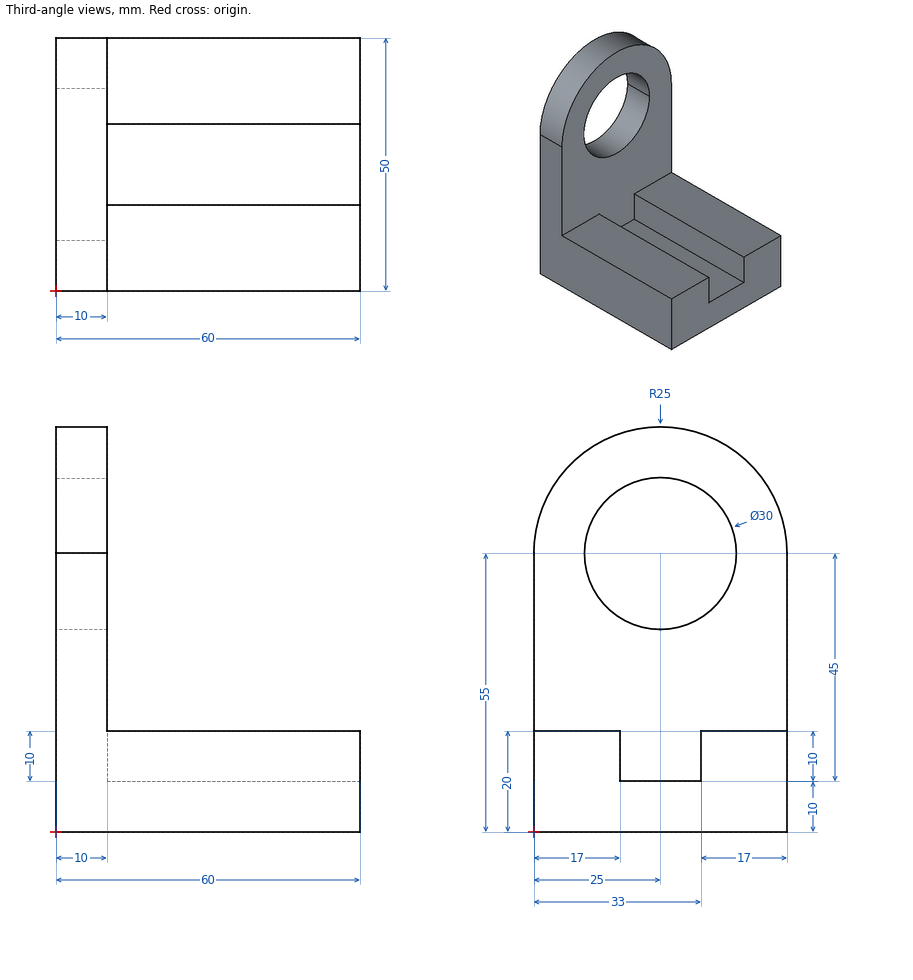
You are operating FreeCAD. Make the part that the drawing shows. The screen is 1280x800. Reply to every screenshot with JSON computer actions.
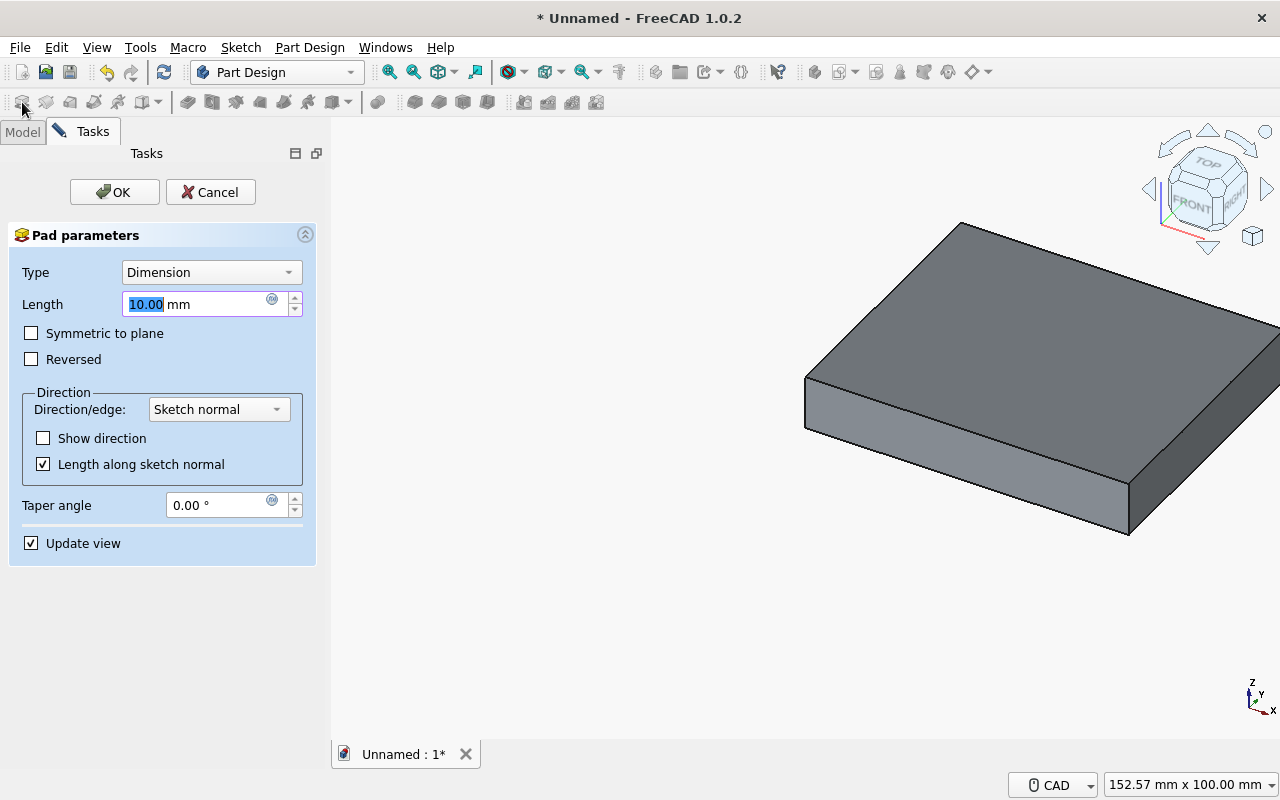
{"action": "type", "text": "60"}
{"action": "key", "text": "Tab"}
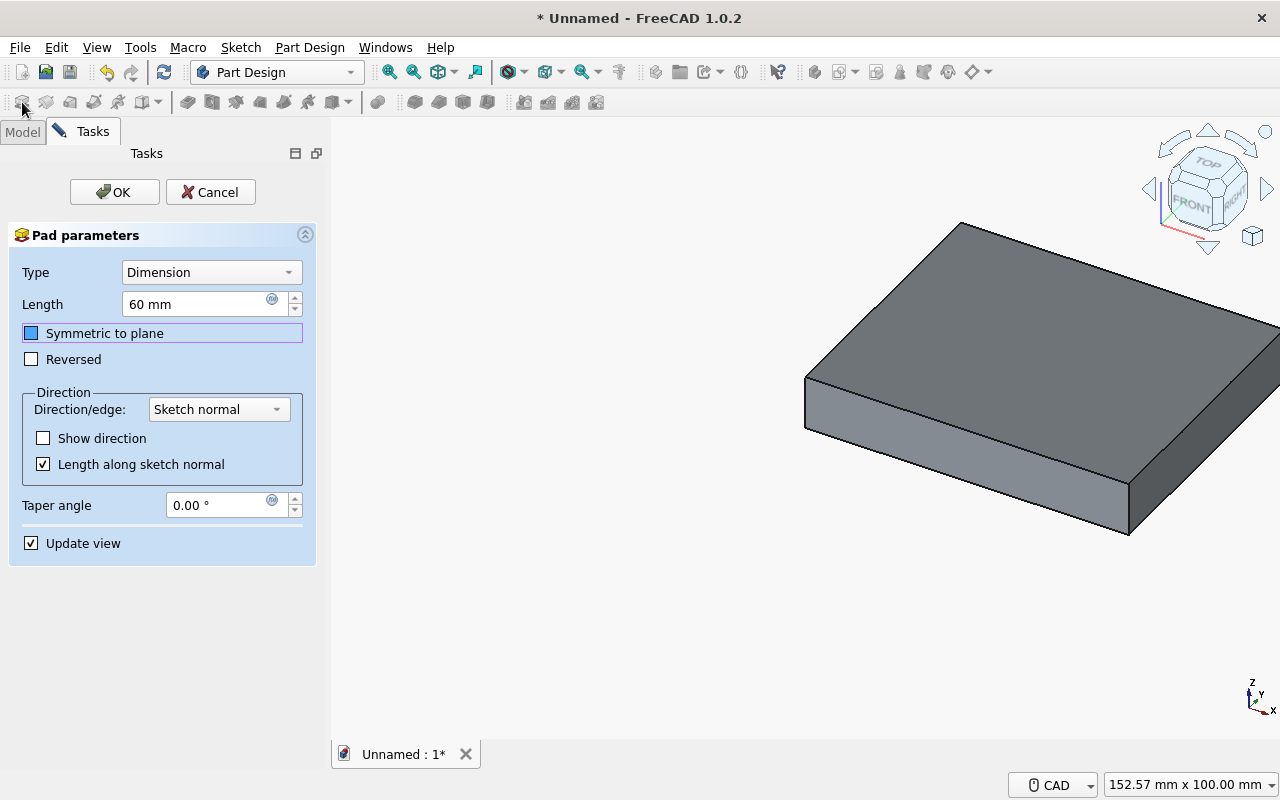
{"action": "left_click", "coordinate": [30, 359]}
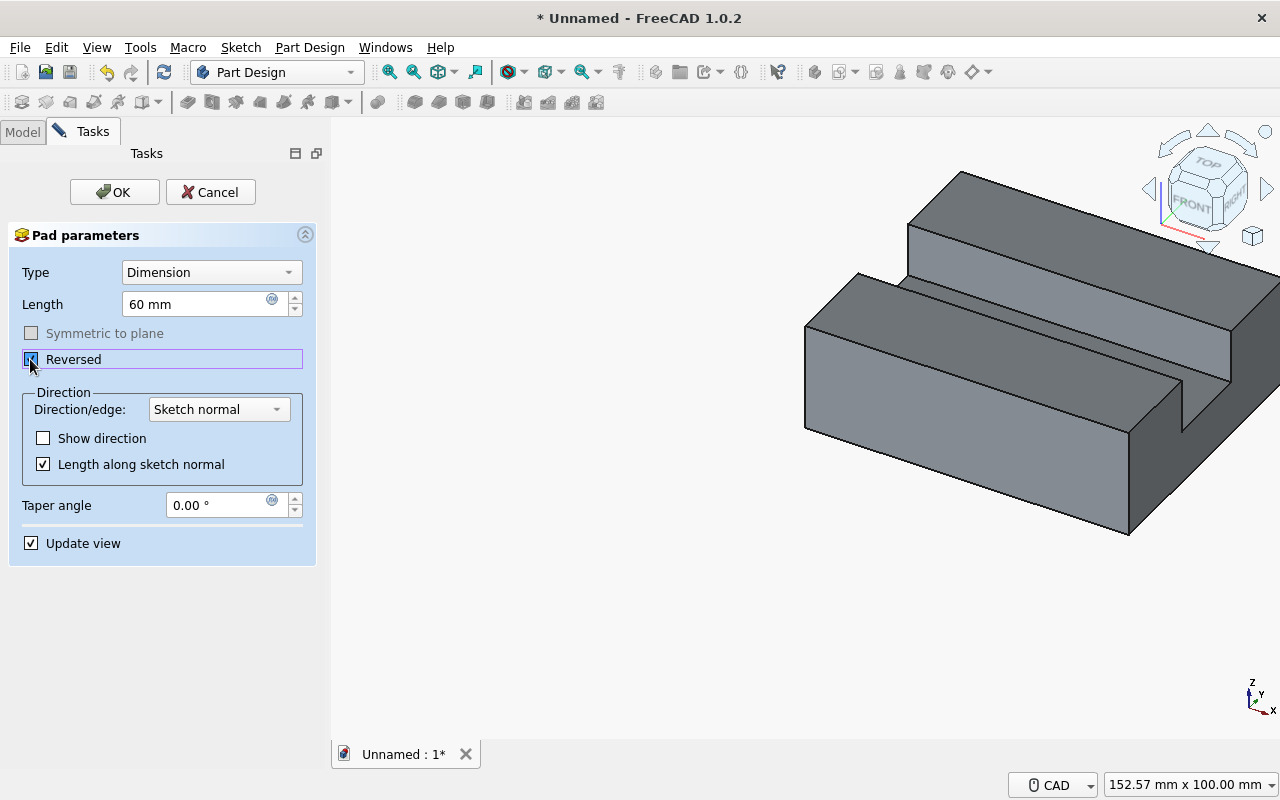
{"action": "left_click", "coordinate": [115, 192]}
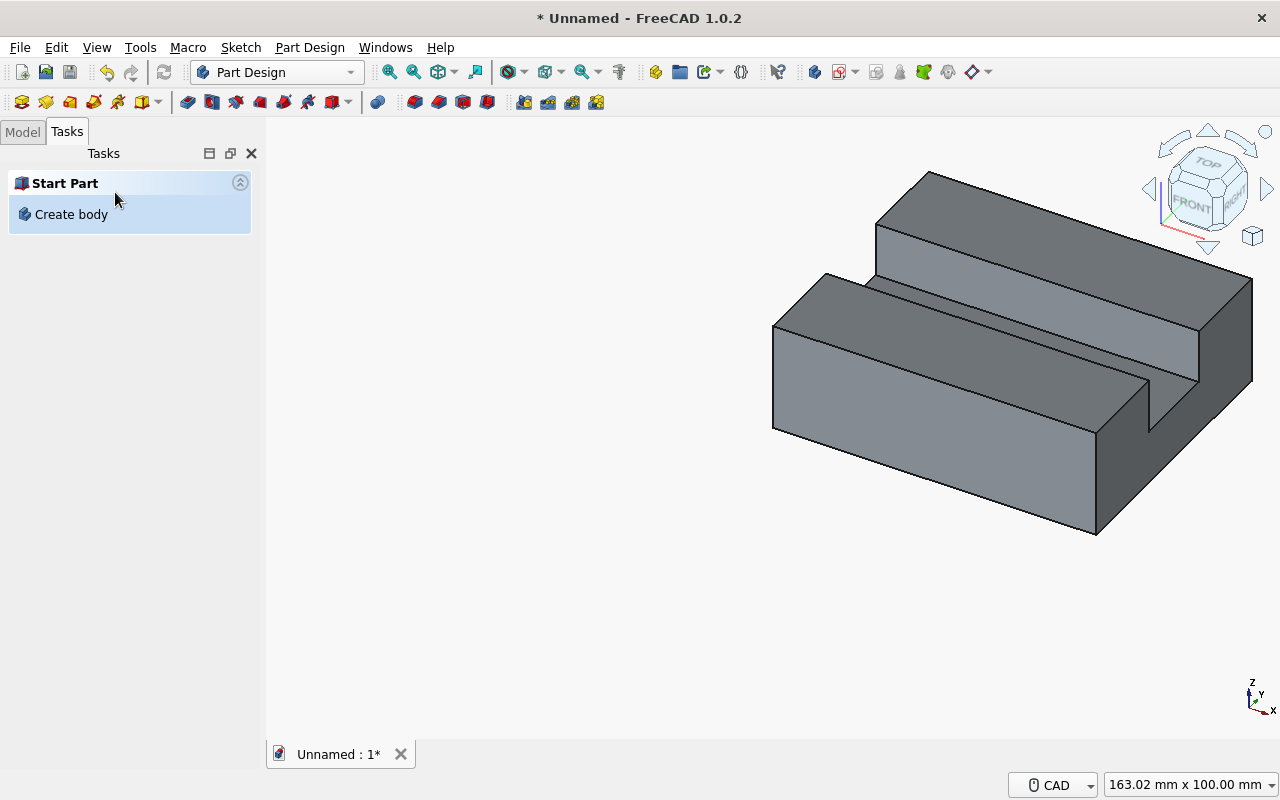
{"action": "left_click", "coordinate": [1053, 383]}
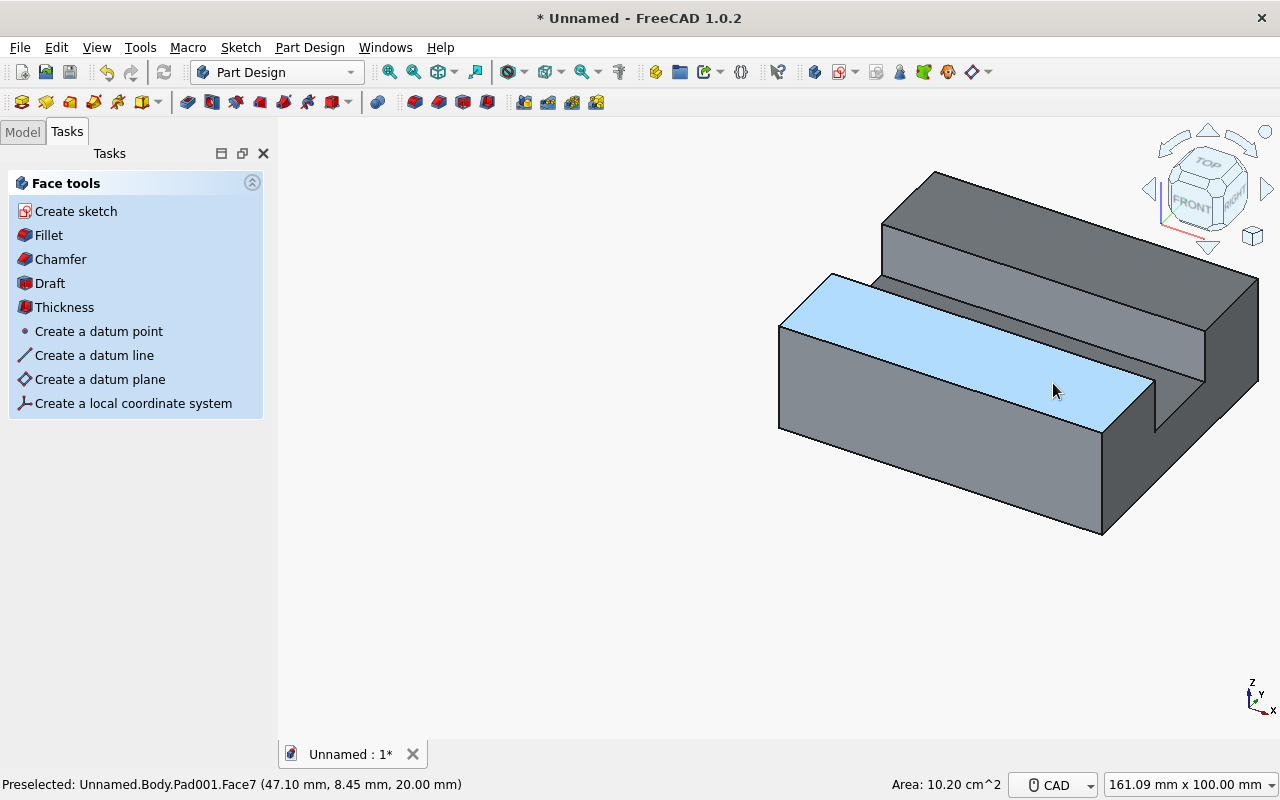
{"action": "left_click", "coordinate": [840, 72]}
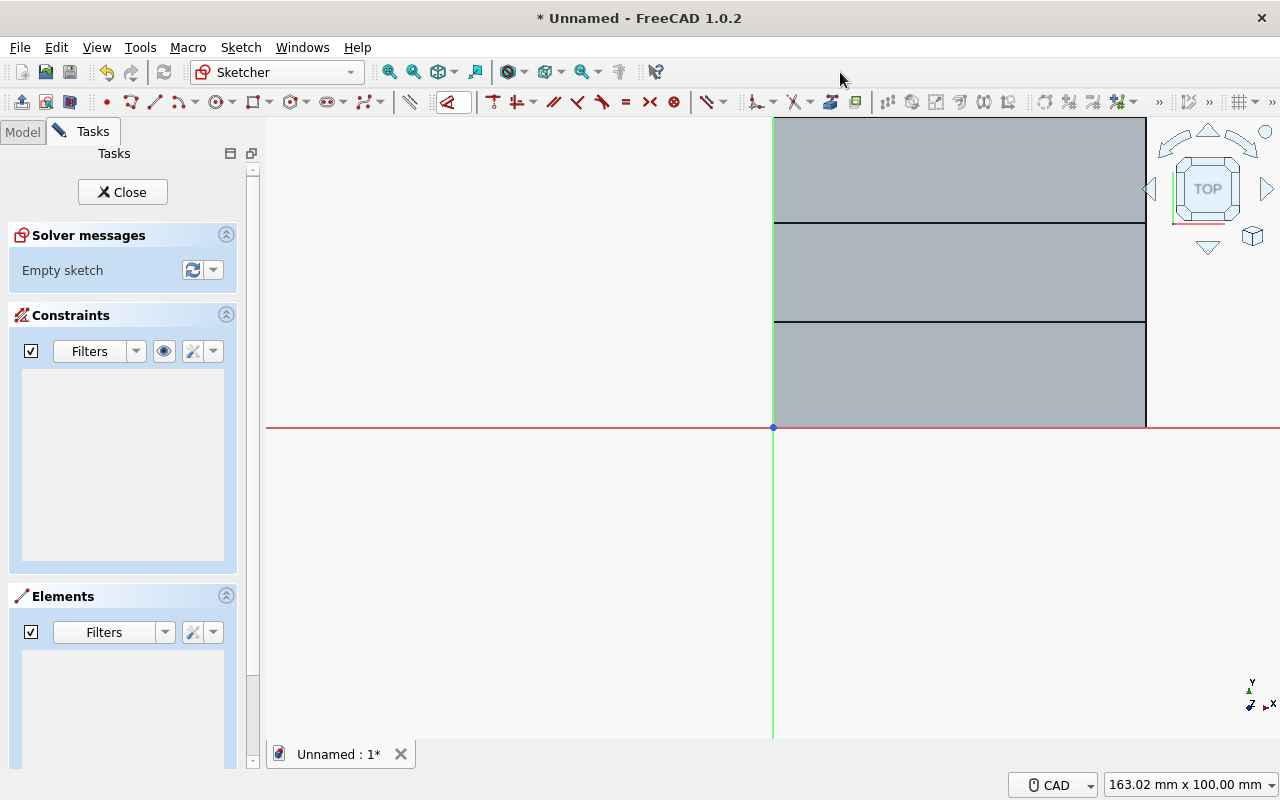
{"action": "scroll", "coordinate": [294, 711], "scroll_direction": "down", "scroll_amount": 1}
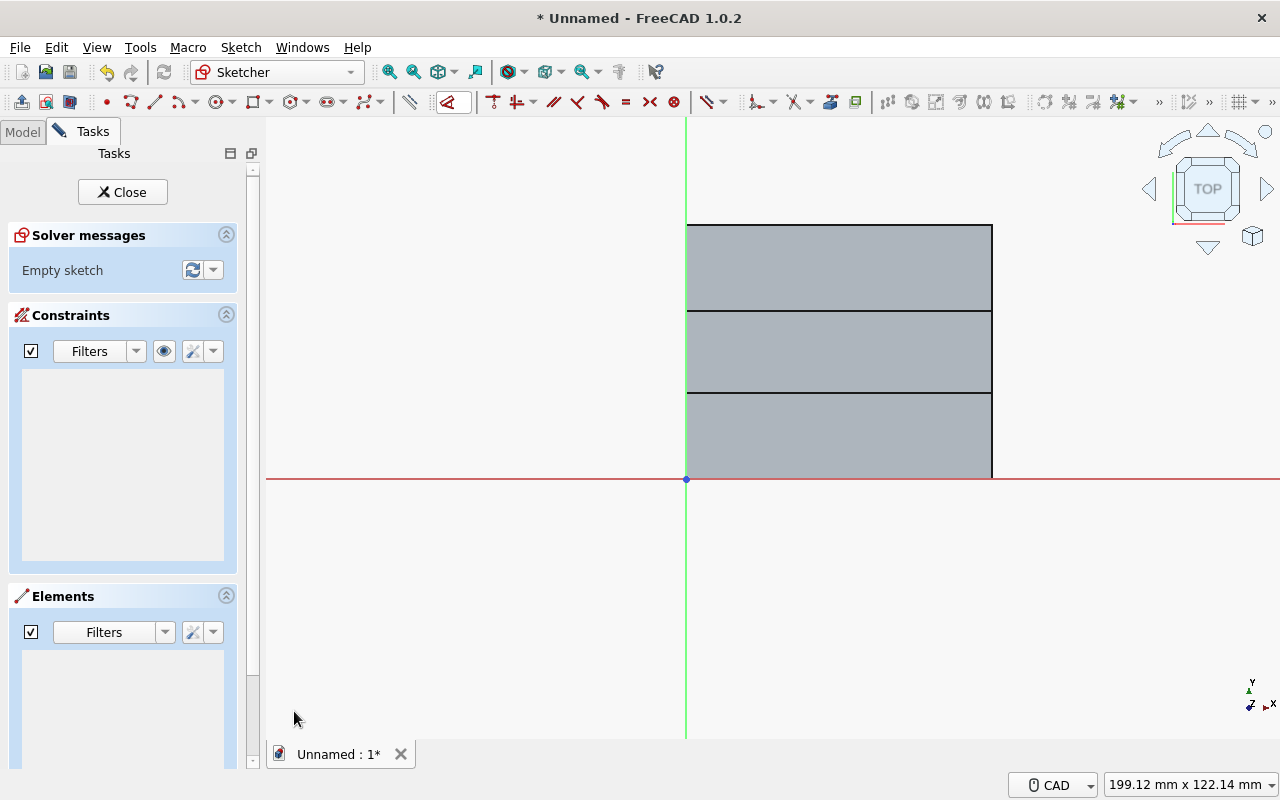
{"action": "scroll", "coordinate": [726, 198], "scroll_direction": "up", "scroll_amount": 2}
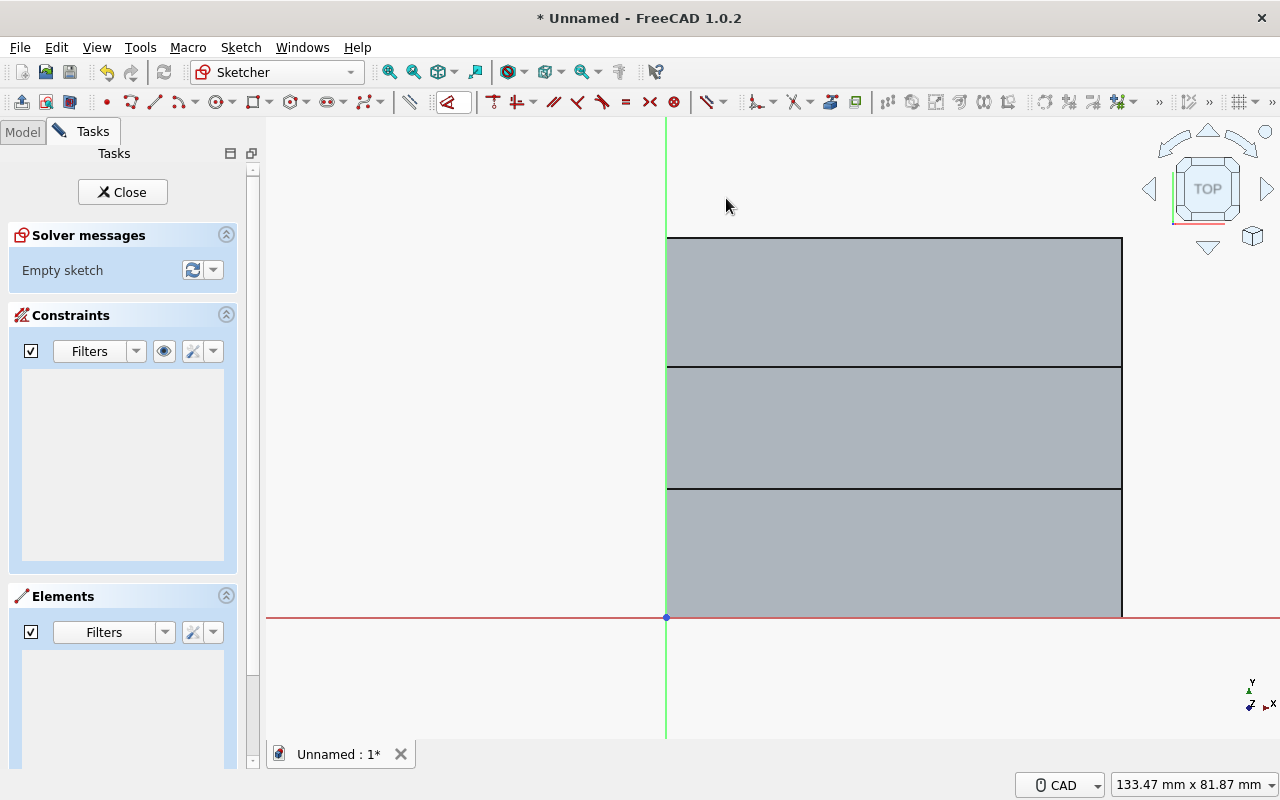
{"action": "left_click", "coordinate": [254, 102]}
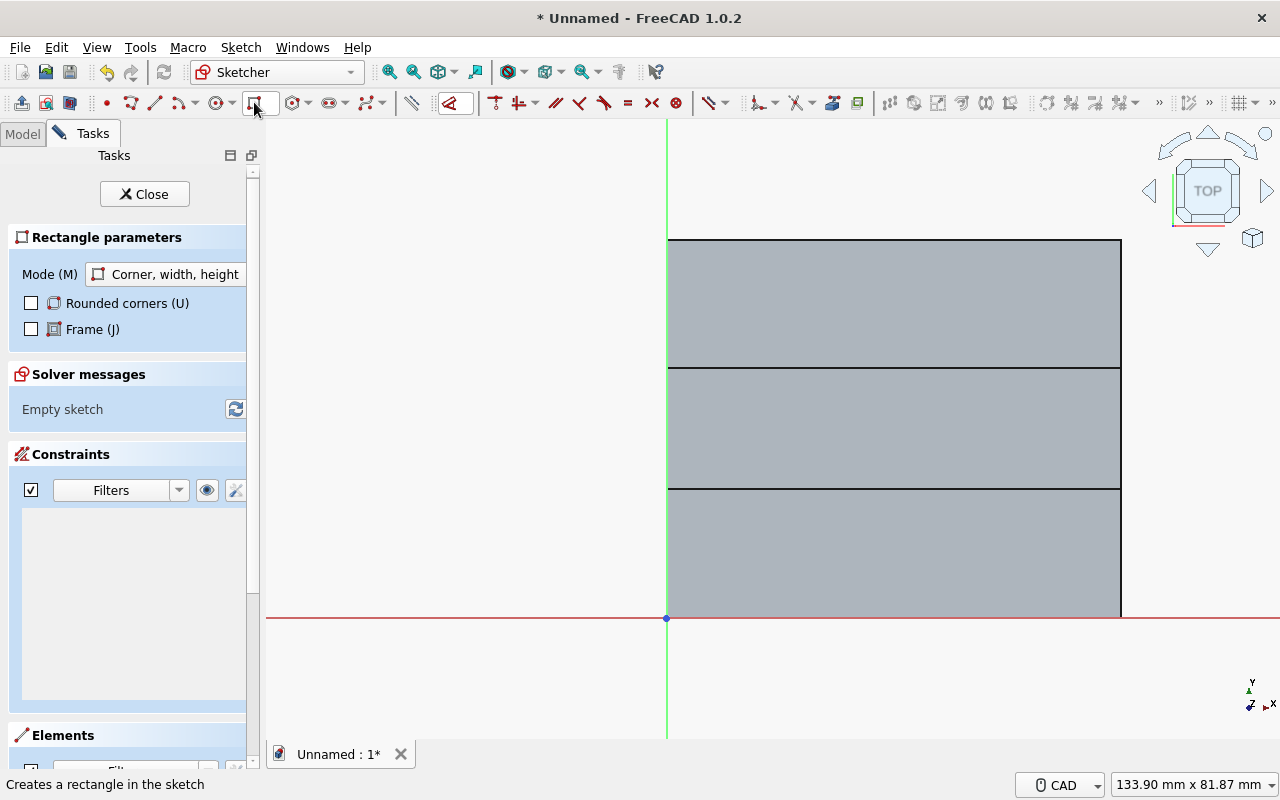
{"action": "left_click", "coordinate": [667, 618]}
{"action": "left_click", "coordinate": [742, 240]}
{"action": "key", "text": "Escape"}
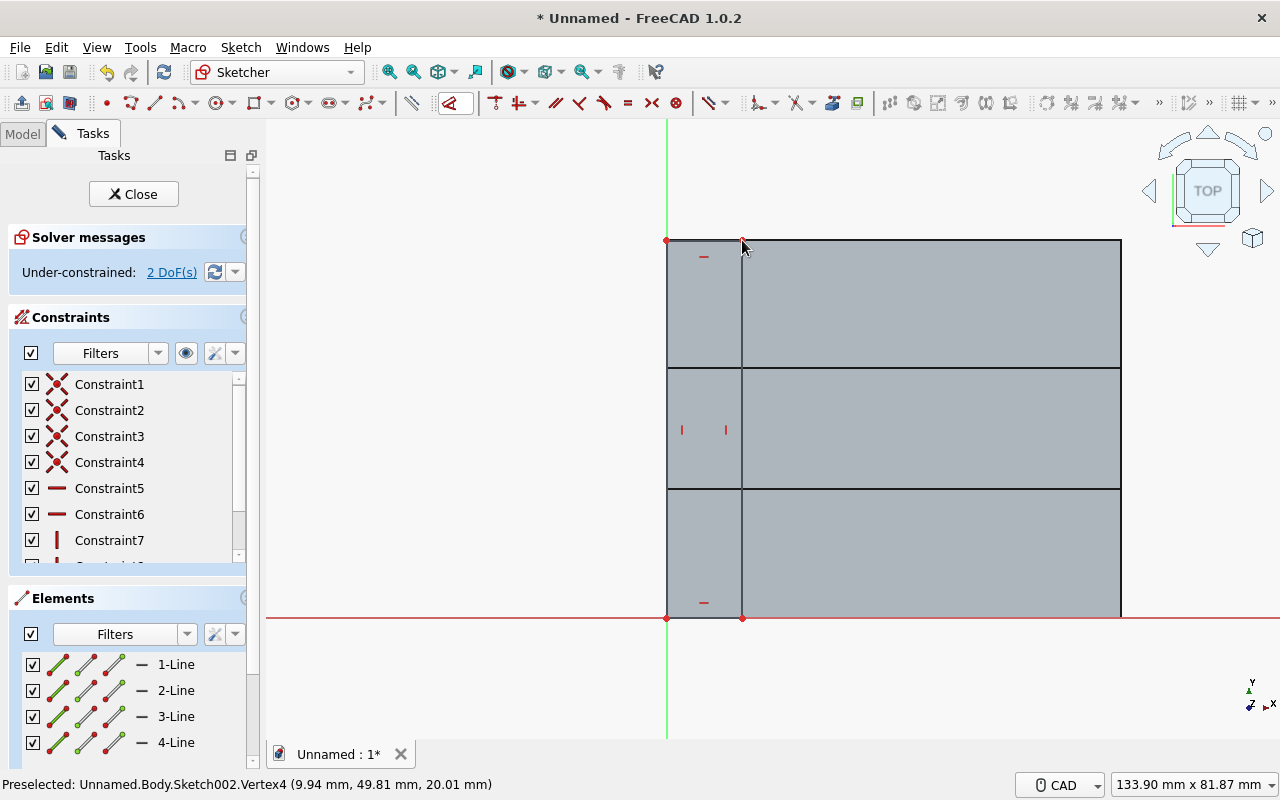
{"action": "left_click", "coordinate": [689, 618]}